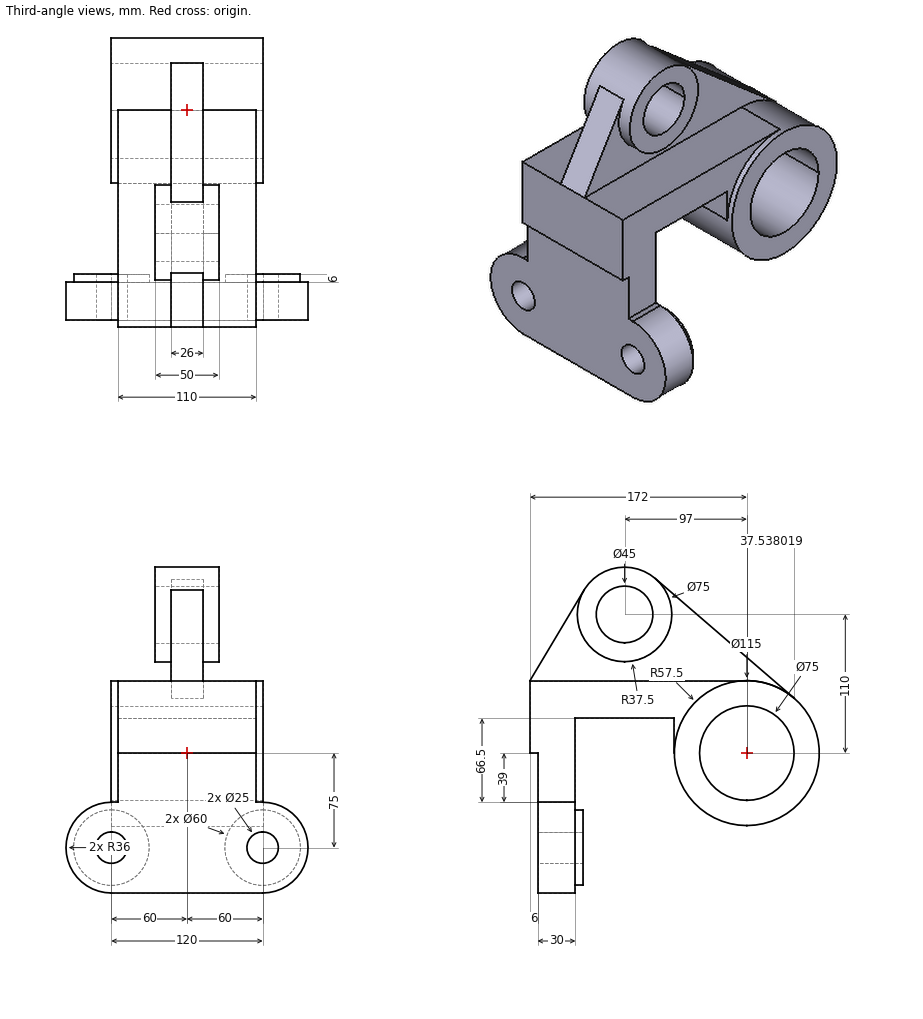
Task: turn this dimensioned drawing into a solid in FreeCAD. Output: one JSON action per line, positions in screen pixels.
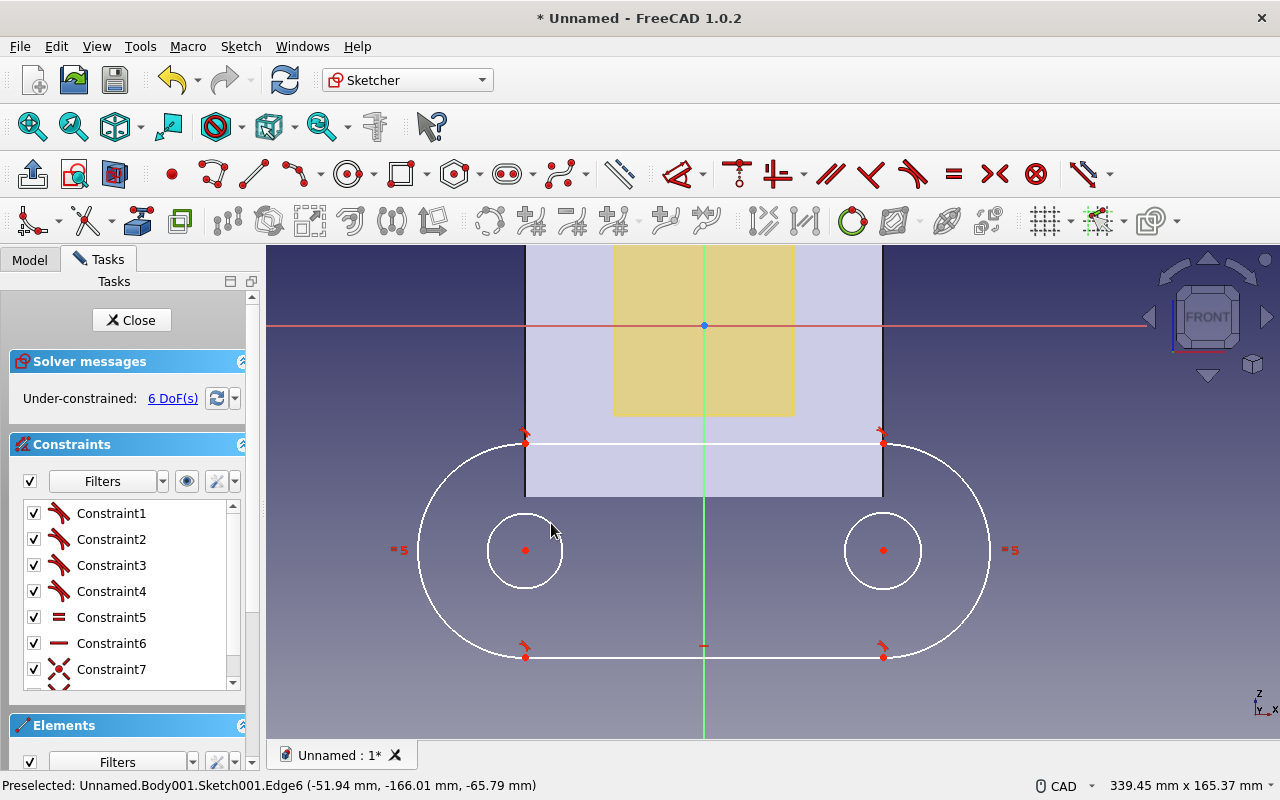
{"action": "left_click", "coordinate": [910, 524]}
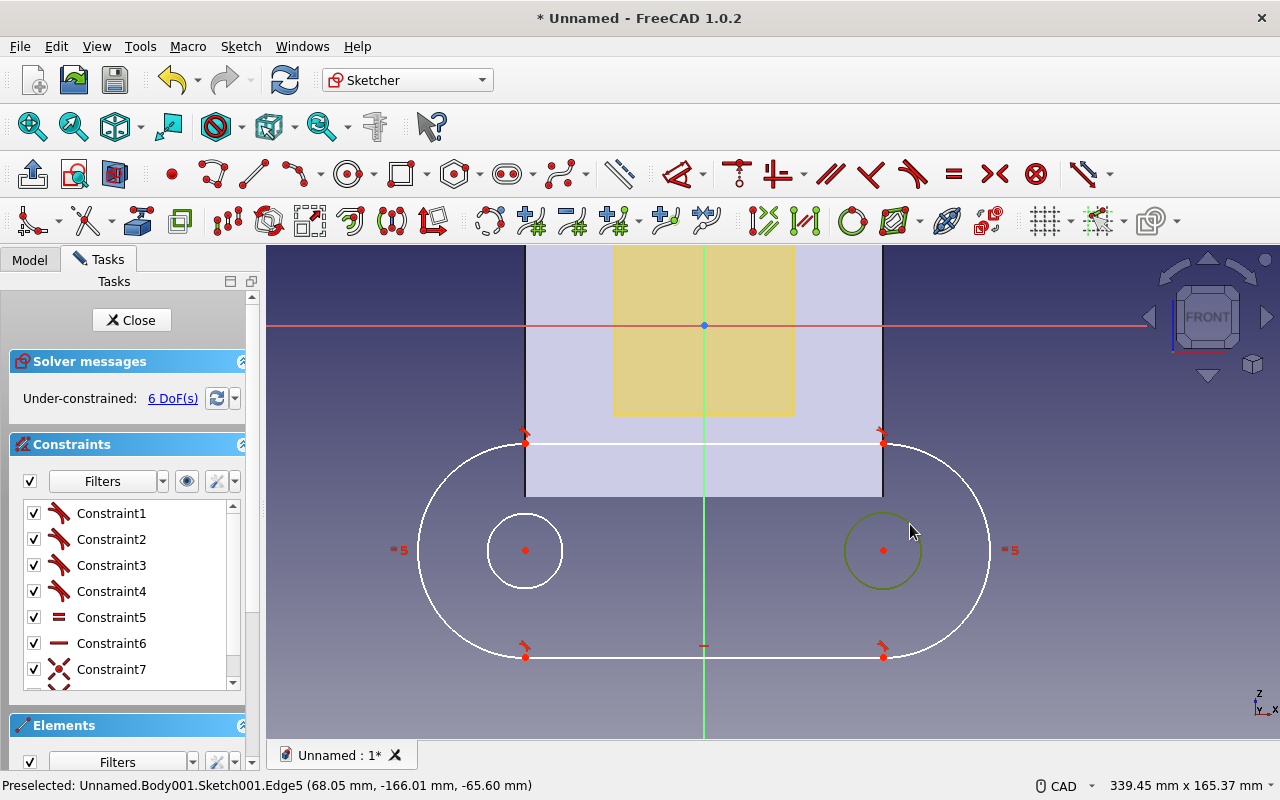
{"action": "left_click", "coordinate": [551, 524]}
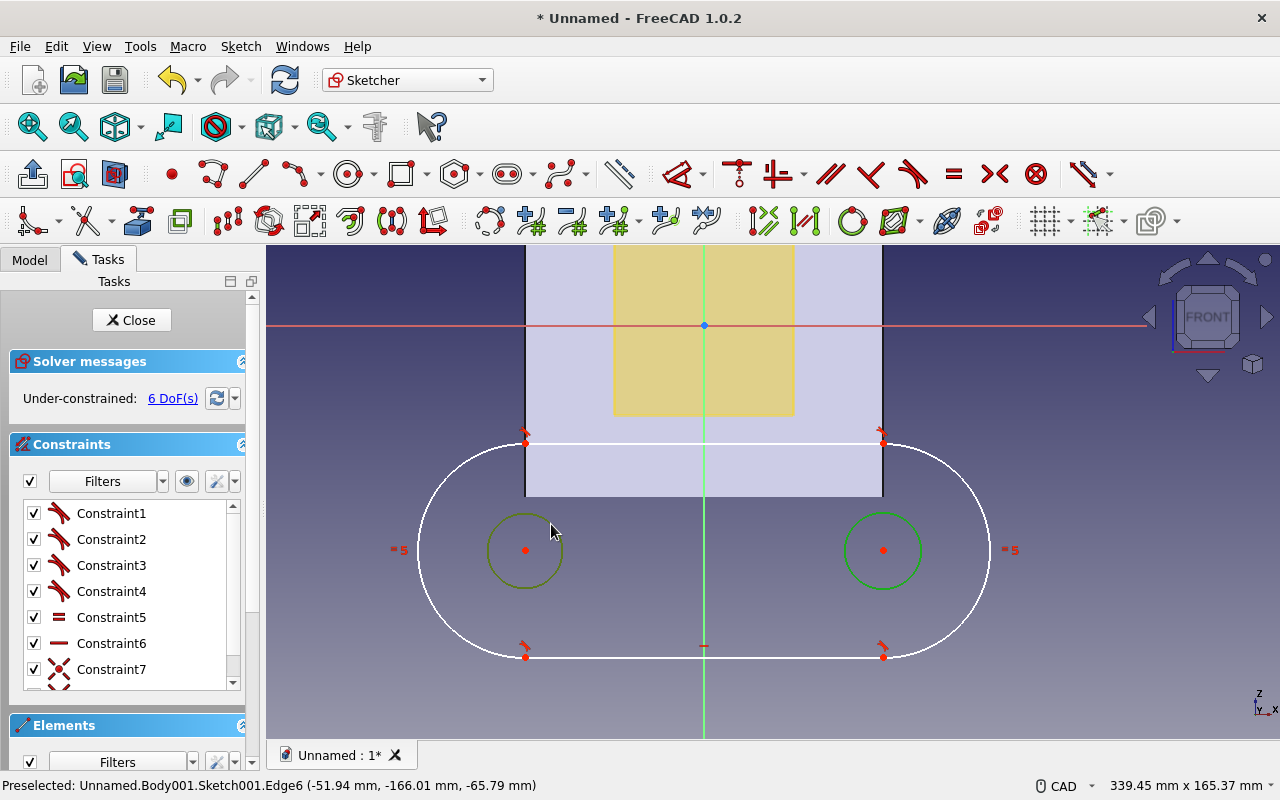
{"action": "left_click", "coordinate": [954, 174]}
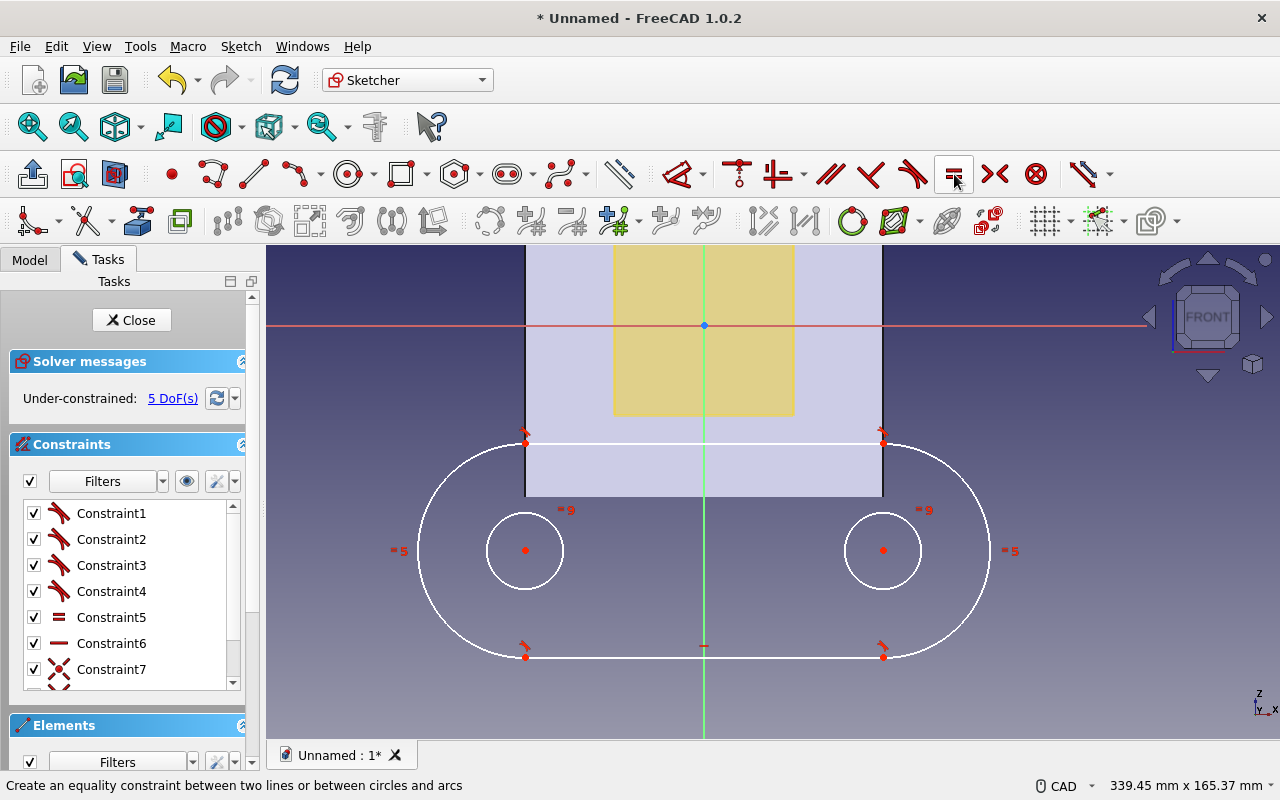
{"action": "key", "text": "d"}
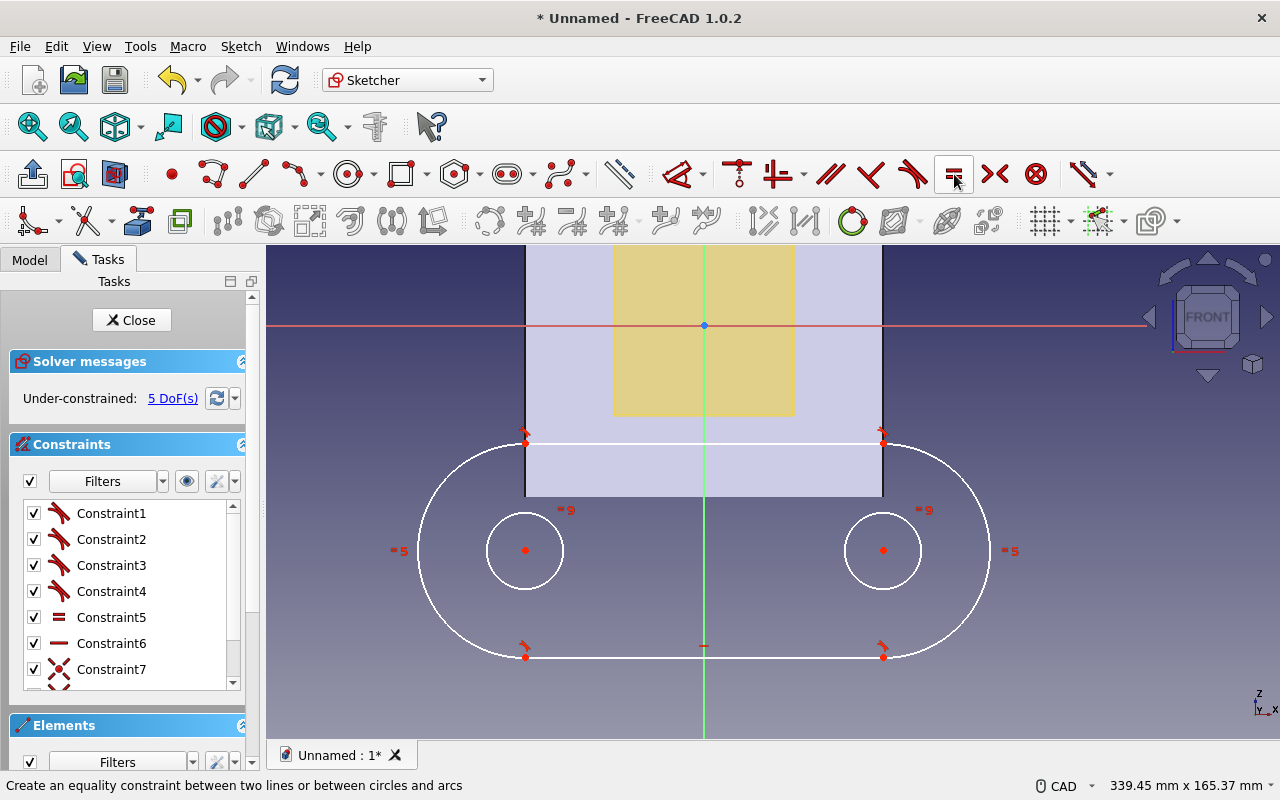
{"action": "left_click", "coordinate": [438, 488]}
{"action": "left_click", "coordinate": [412, 469]}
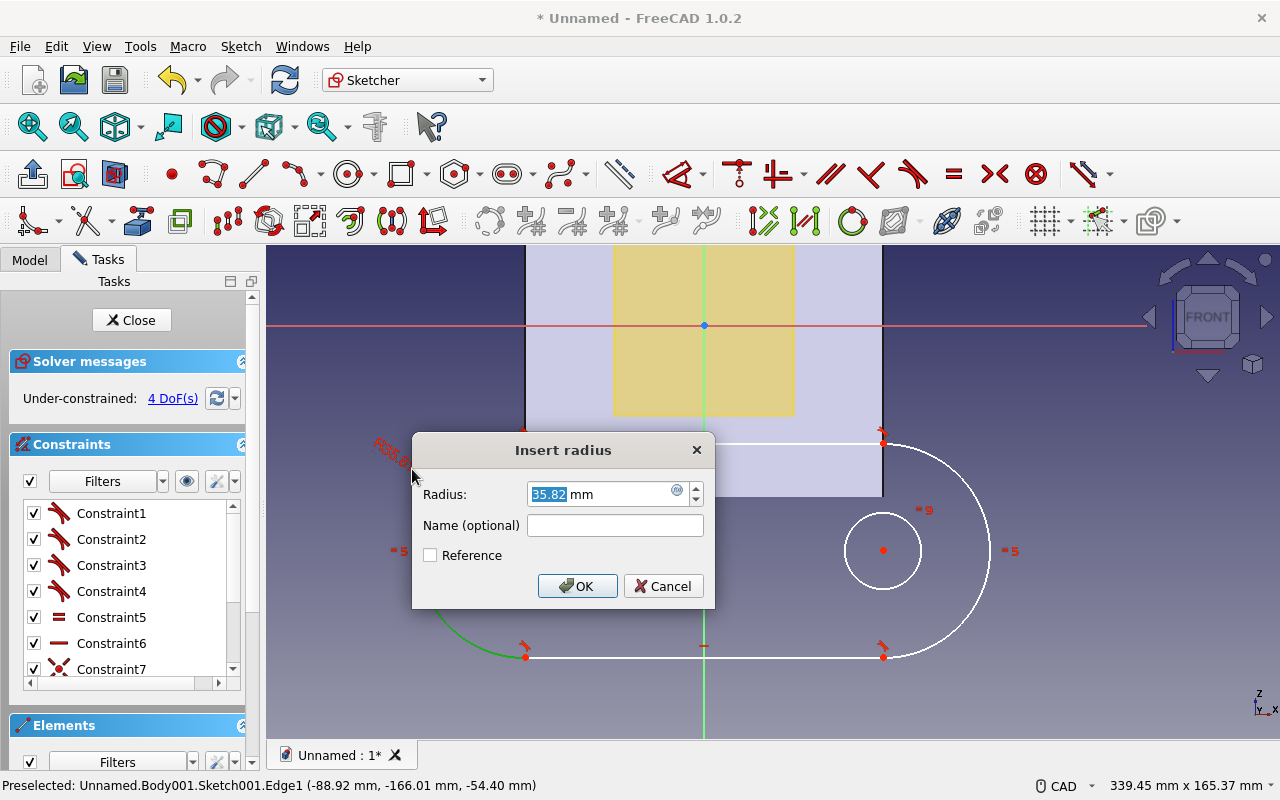
{"action": "type", "text": "36"}
{"action": "key", "text": "Return"}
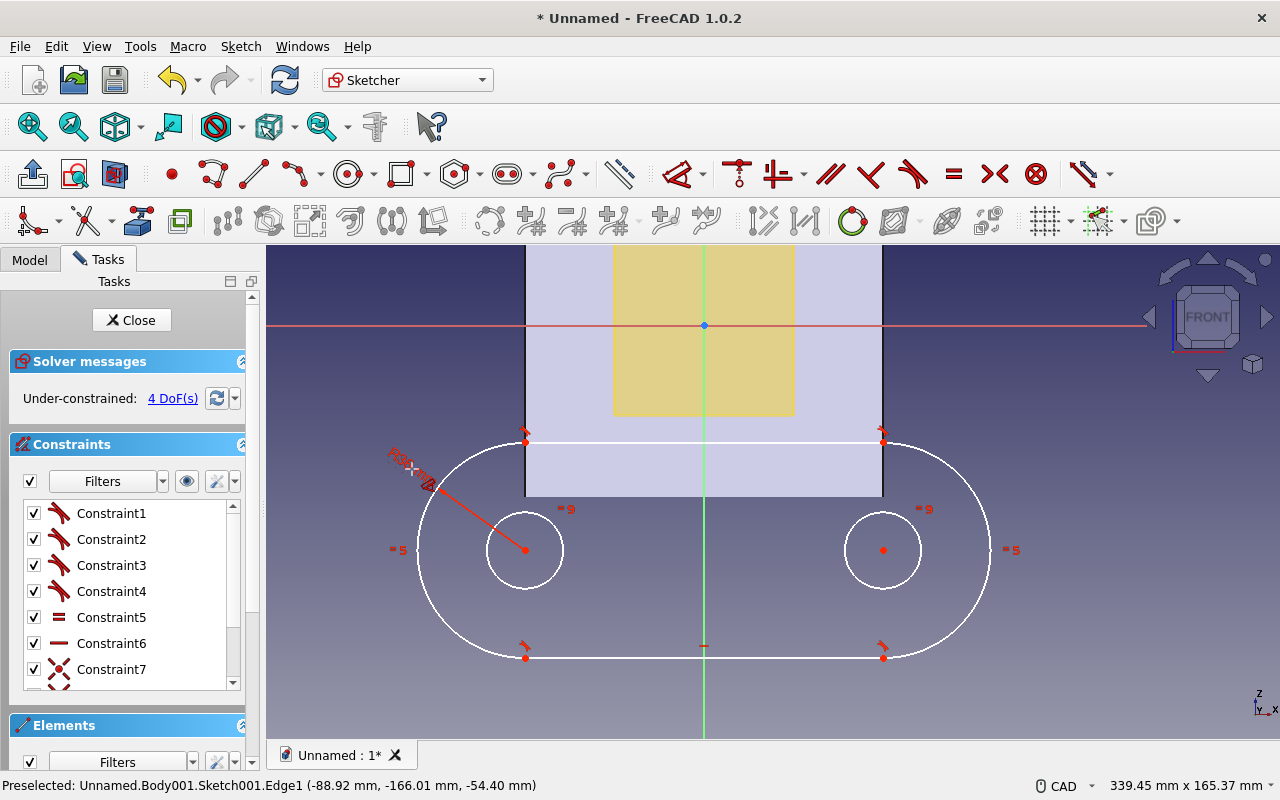
{"action": "left_click", "coordinate": [910, 523]}
{"action": "left_click", "coordinate": [932, 500]}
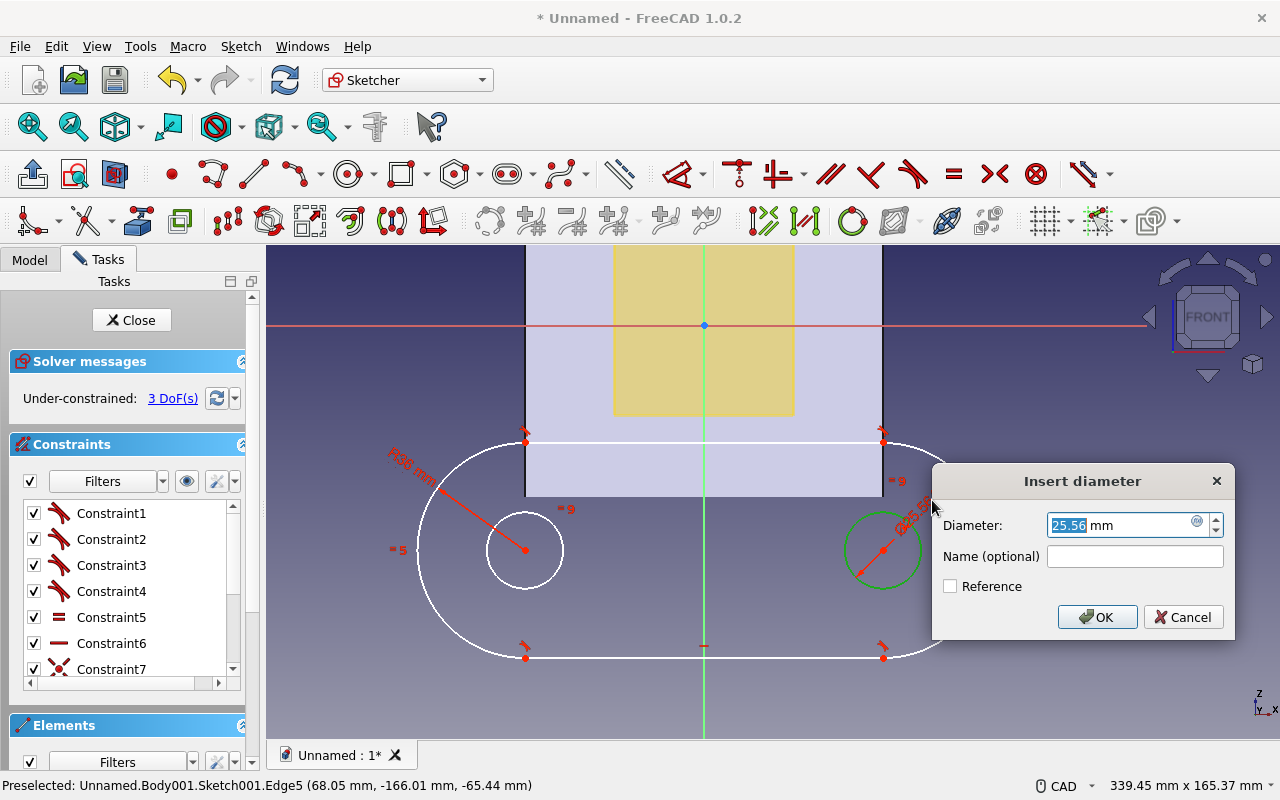
{"action": "type", "text": "25"}
{"action": "key", "text": "Return"}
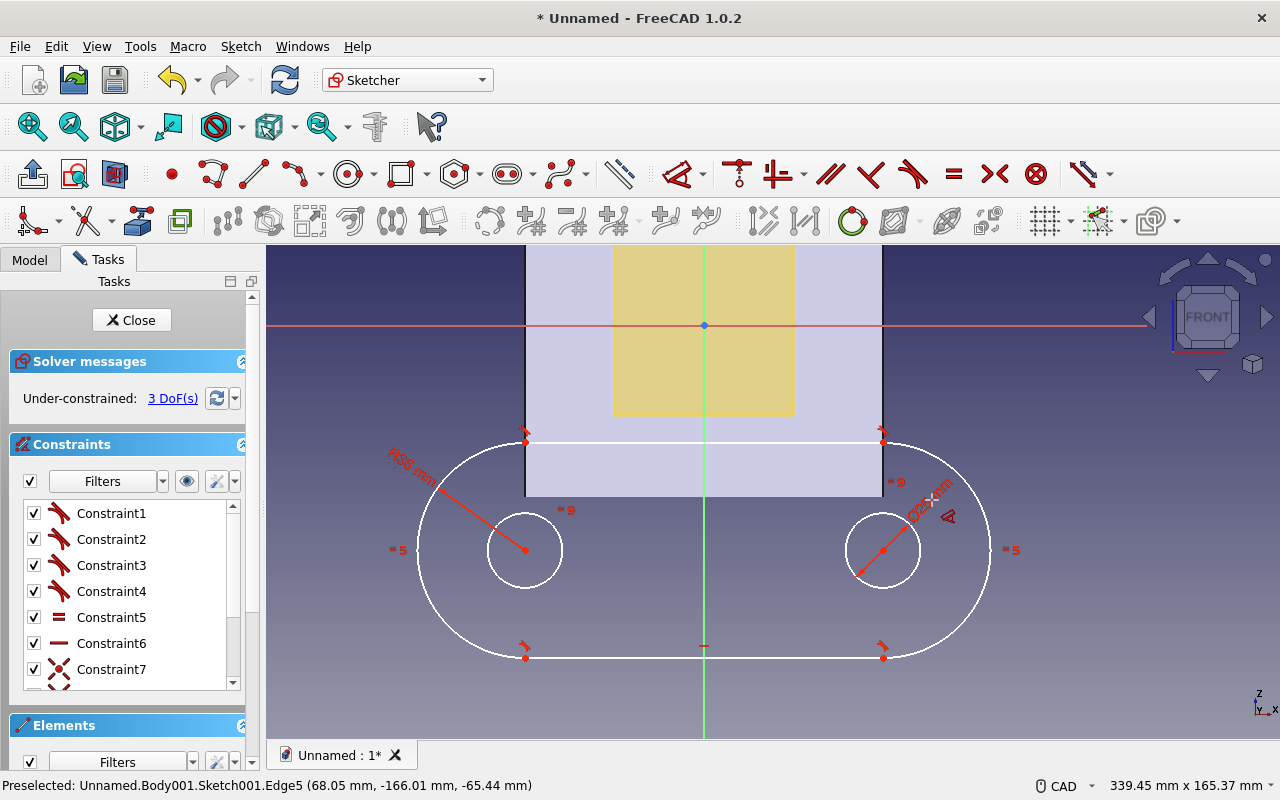
{"action": "left_click", "coordinate": [883, 551]}
{"action": "left_click", "coordinate": [794, 292]}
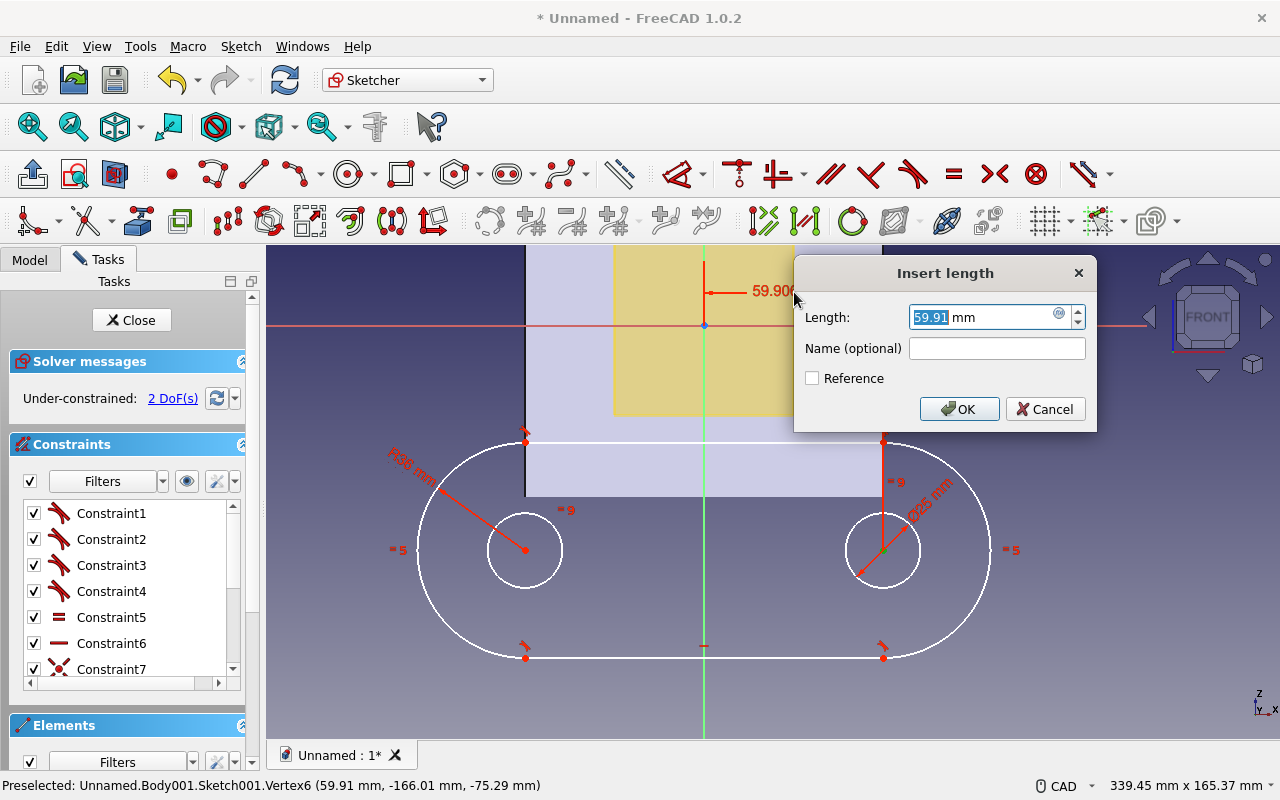
{"action": "type", "text": "60"}
{"action": "key", "text": "Return"}